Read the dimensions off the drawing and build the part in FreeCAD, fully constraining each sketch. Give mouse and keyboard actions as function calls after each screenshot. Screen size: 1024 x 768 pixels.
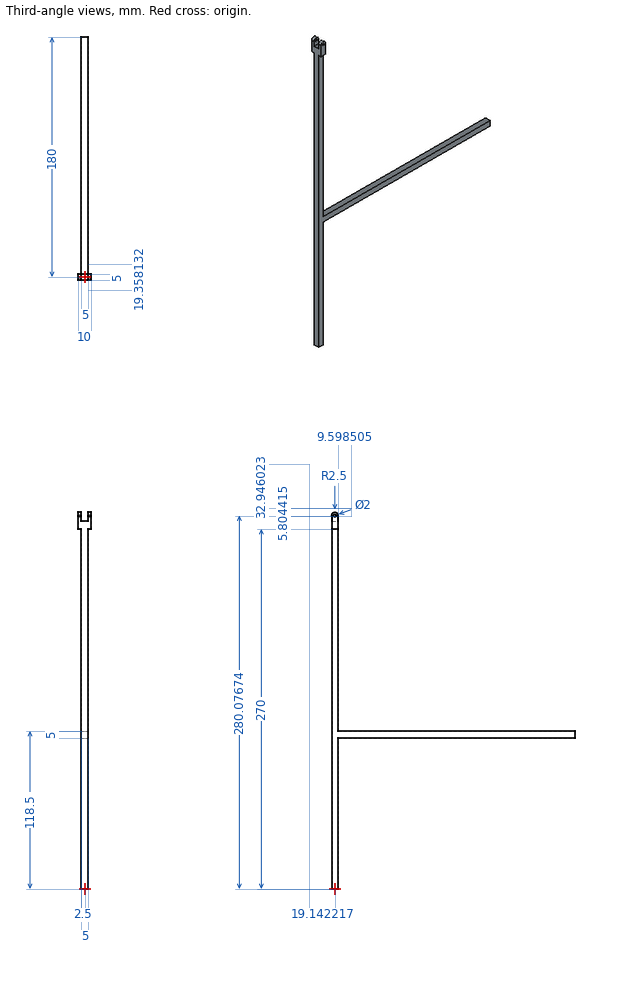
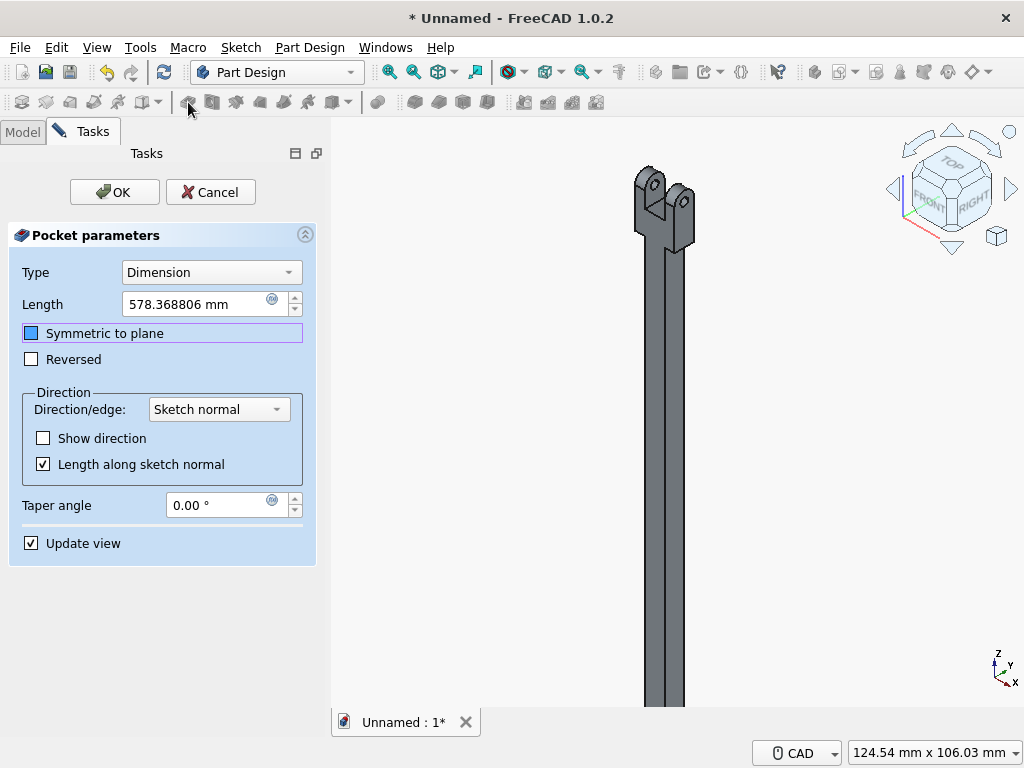
click(30, 333)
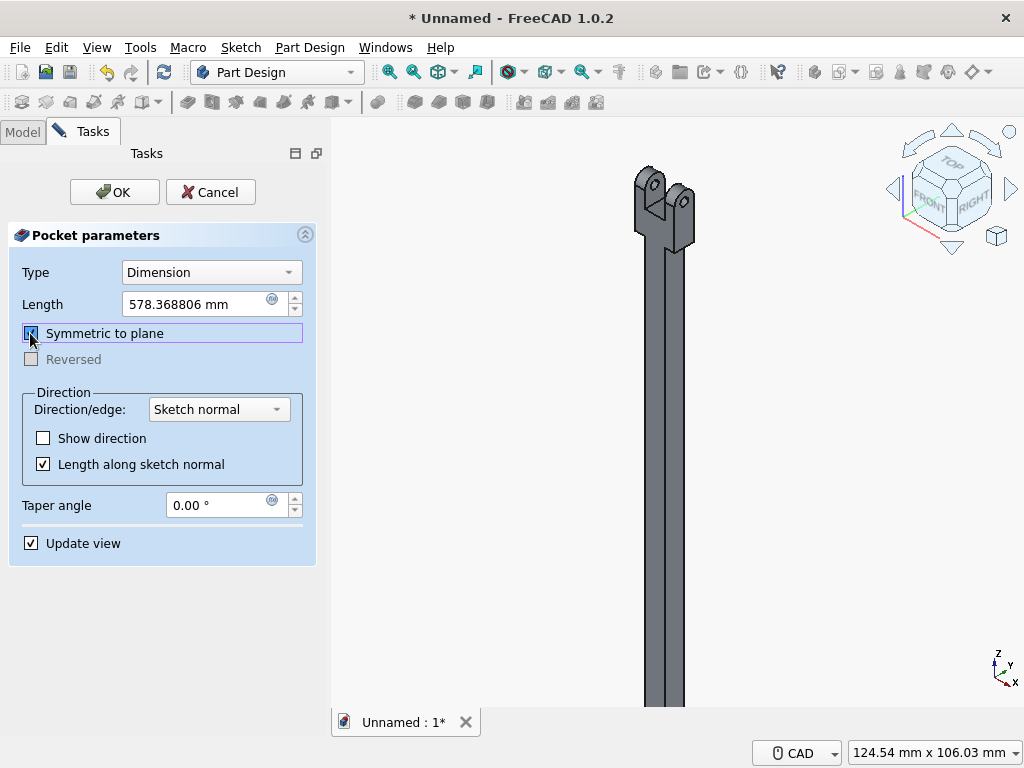
click(115, 192)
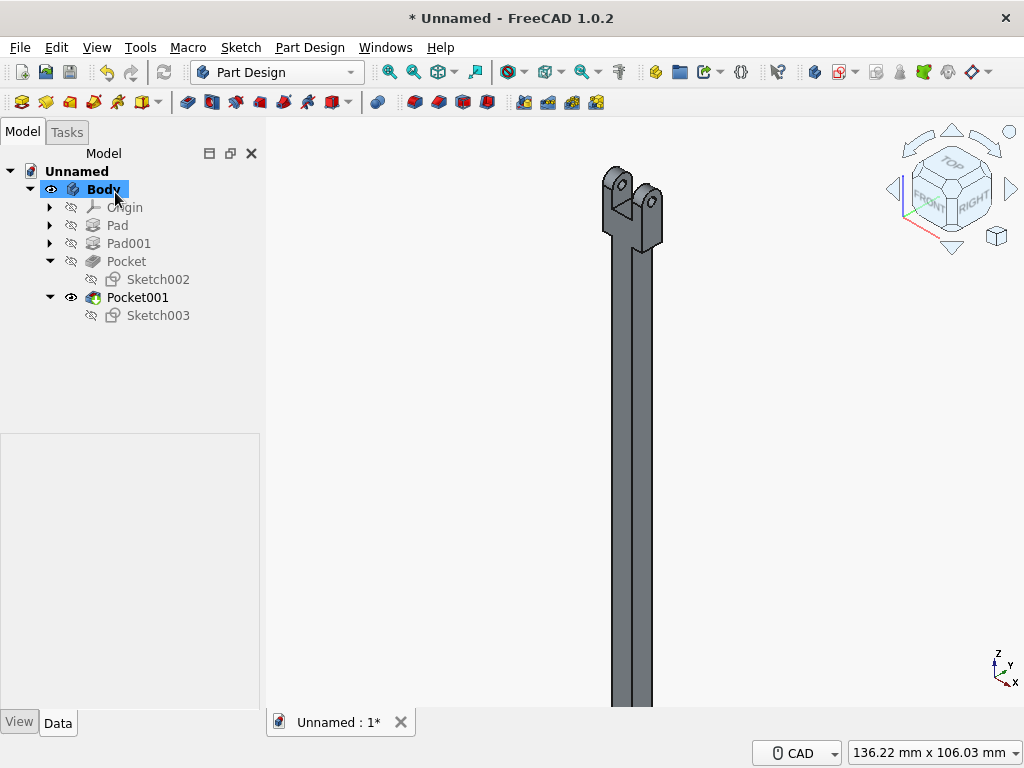
click(390, 72)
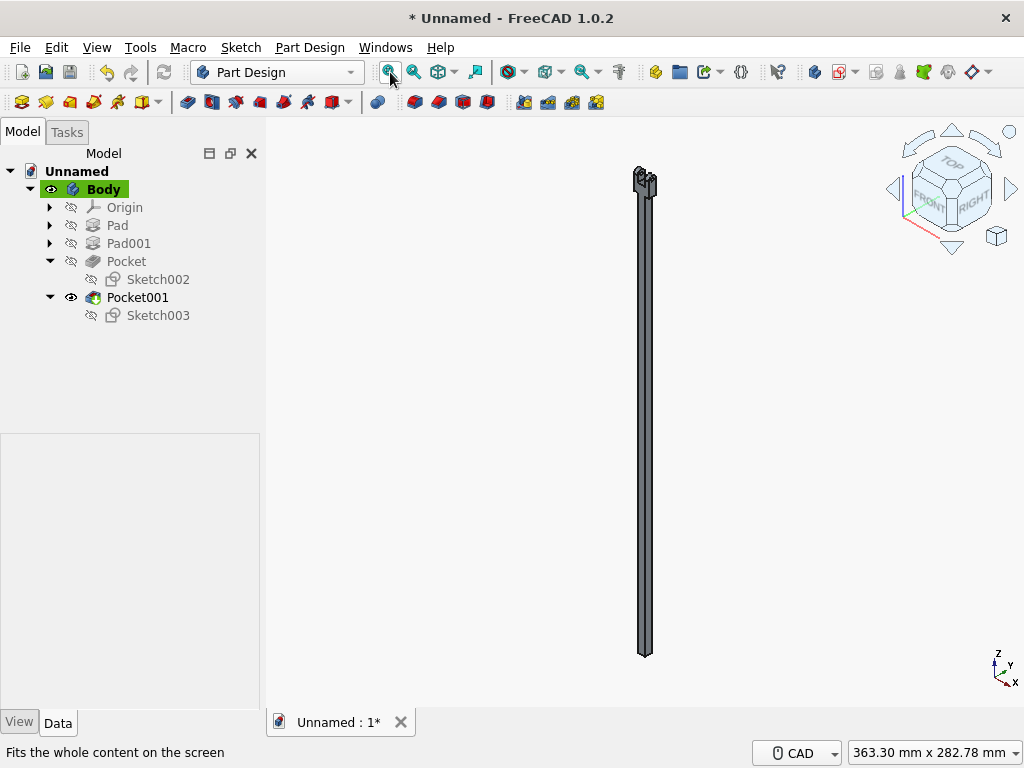
click(840, 72)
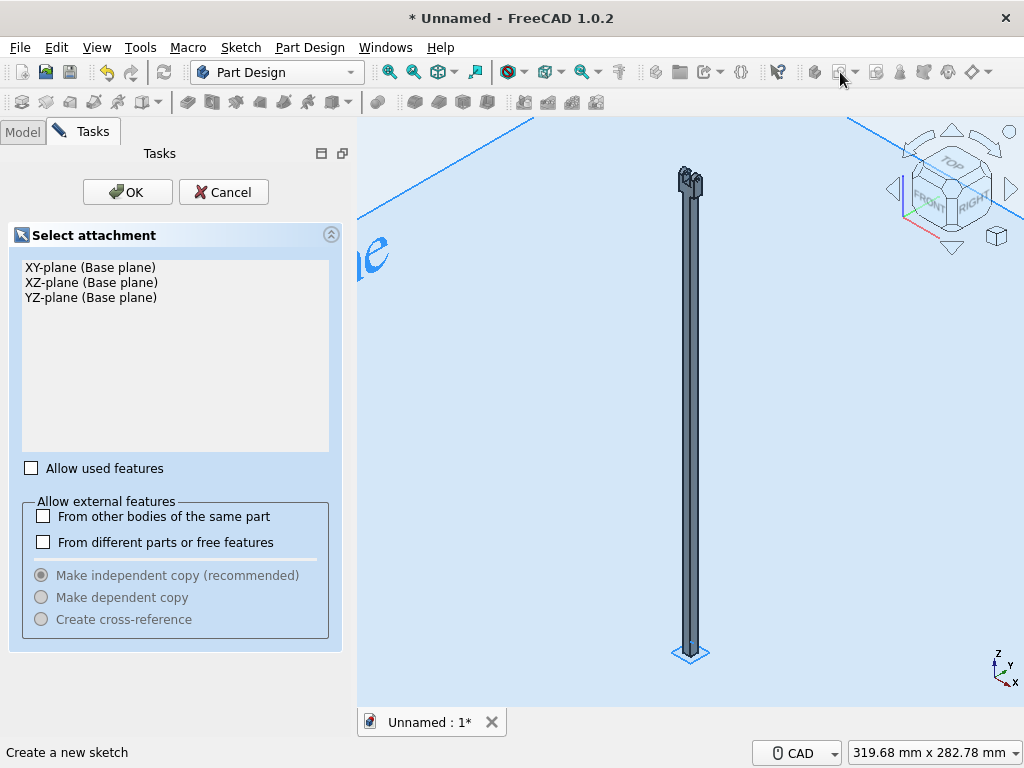
click(82, 282)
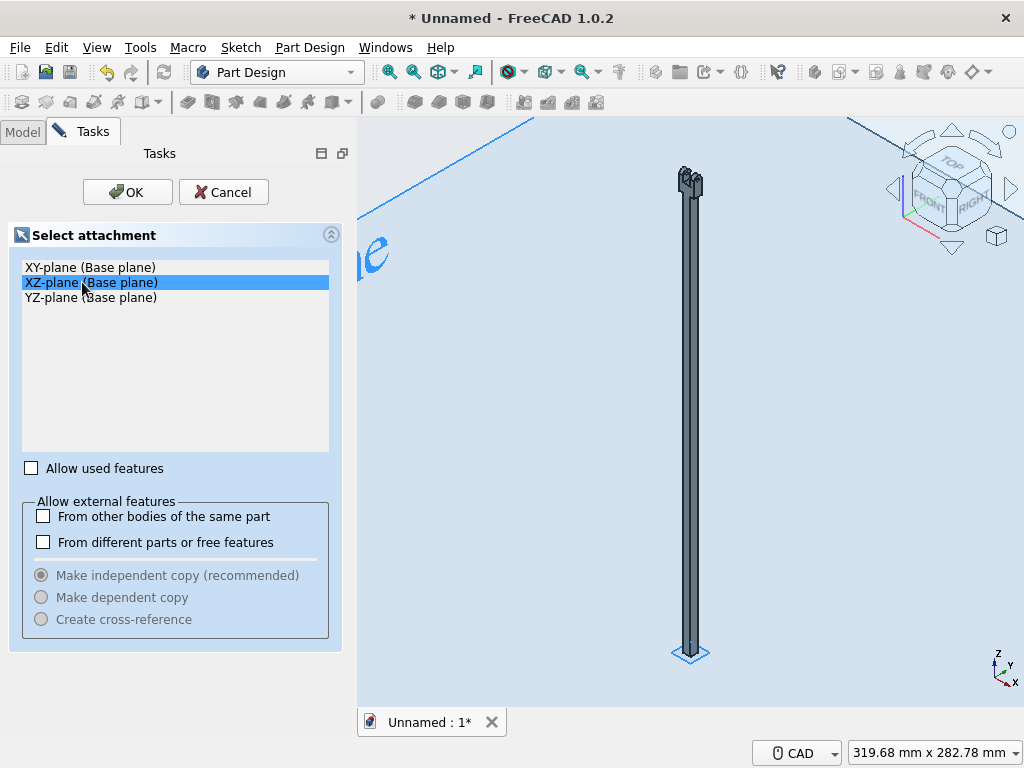
click(128, 192)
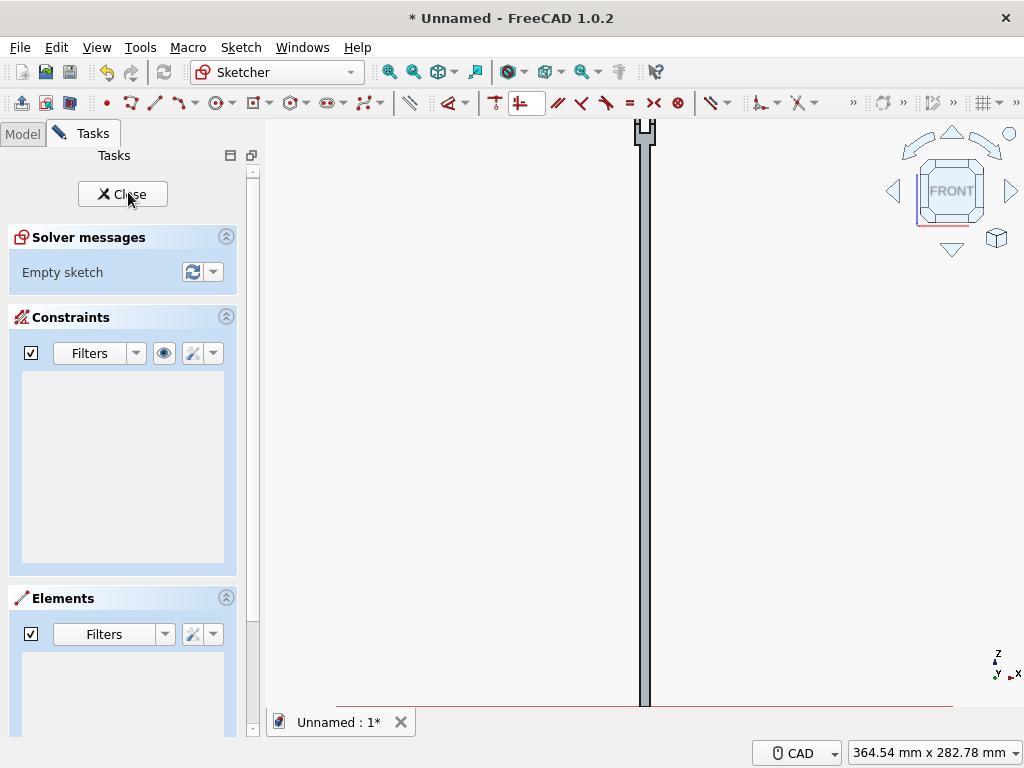
click(70, 104)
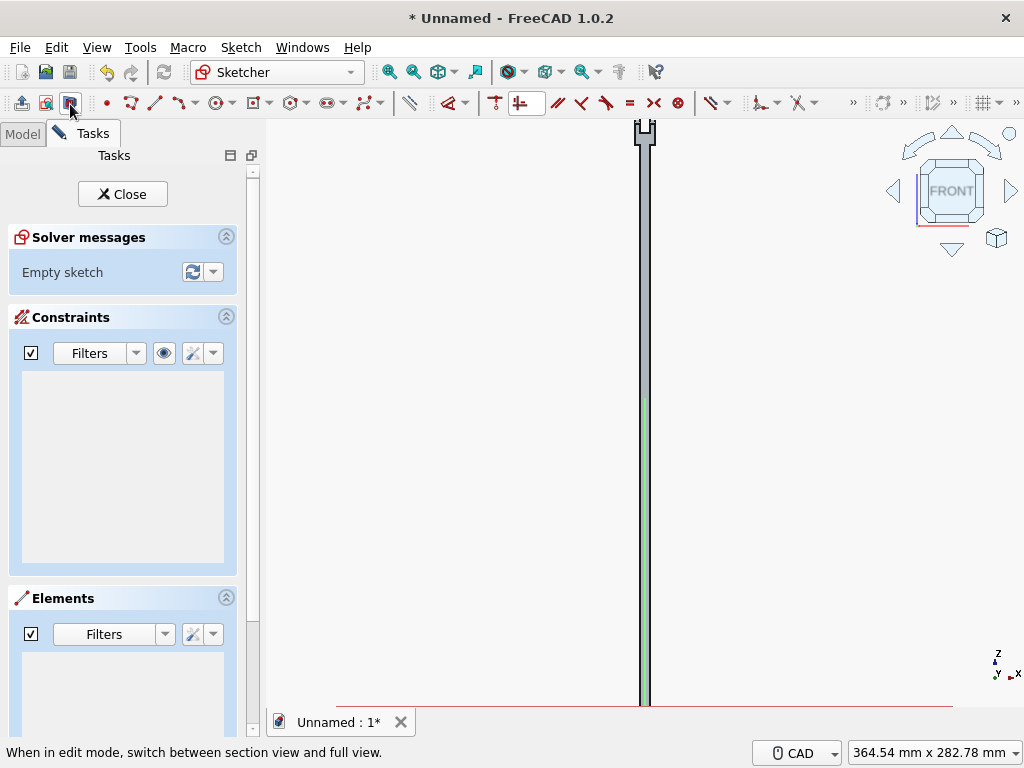
scroll(649, 468, up, 15)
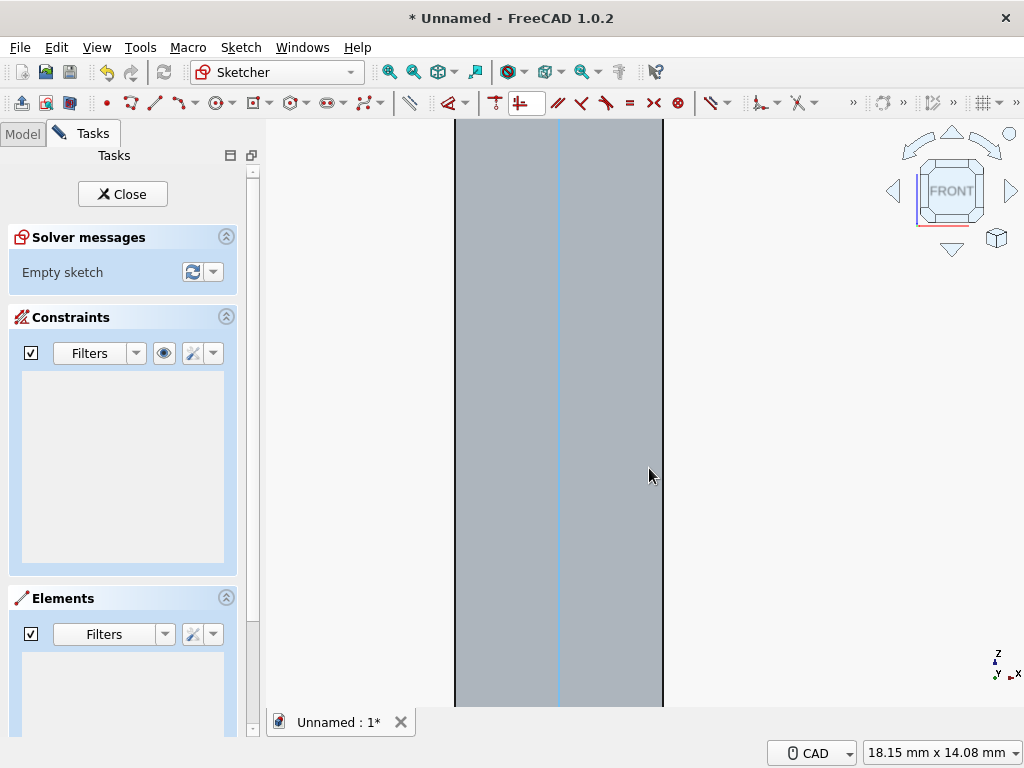
scroll(538, 401, up, 3)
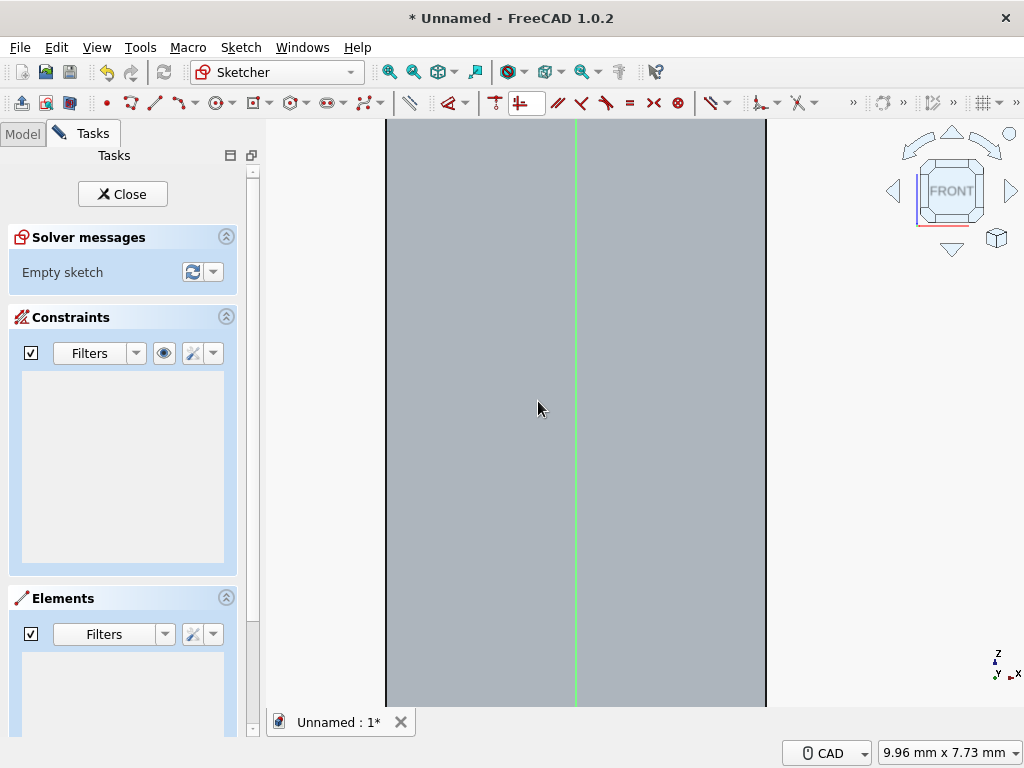
key(g)
key(r)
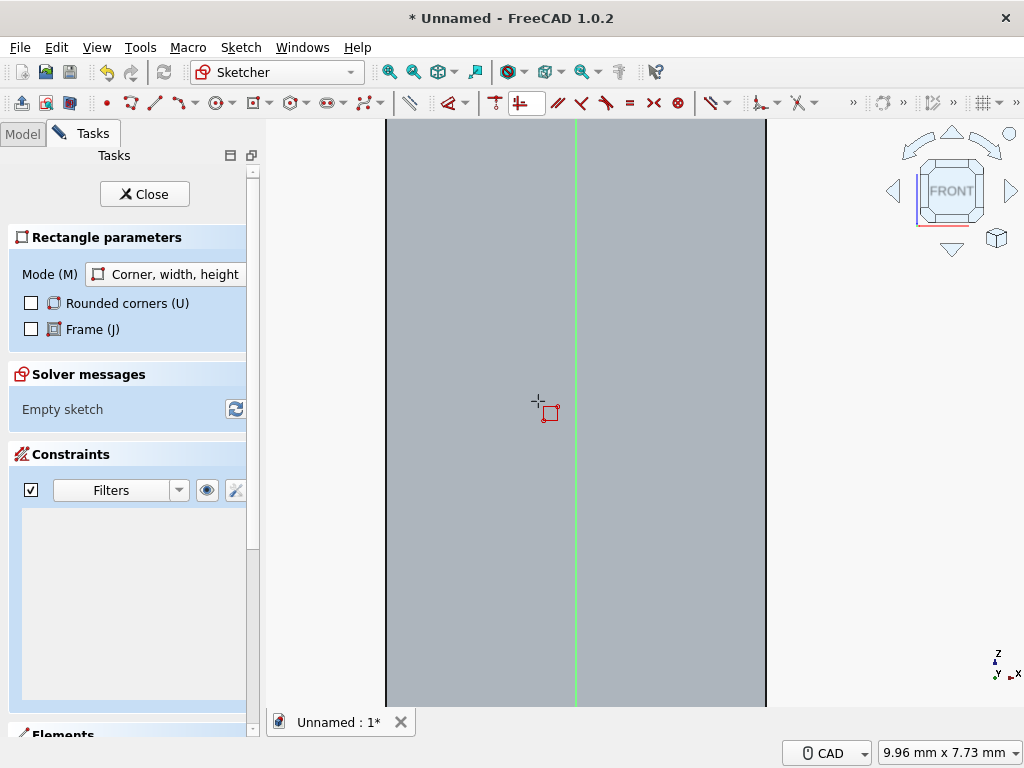
click(386, 223)
click(766, 603)
key(Escape)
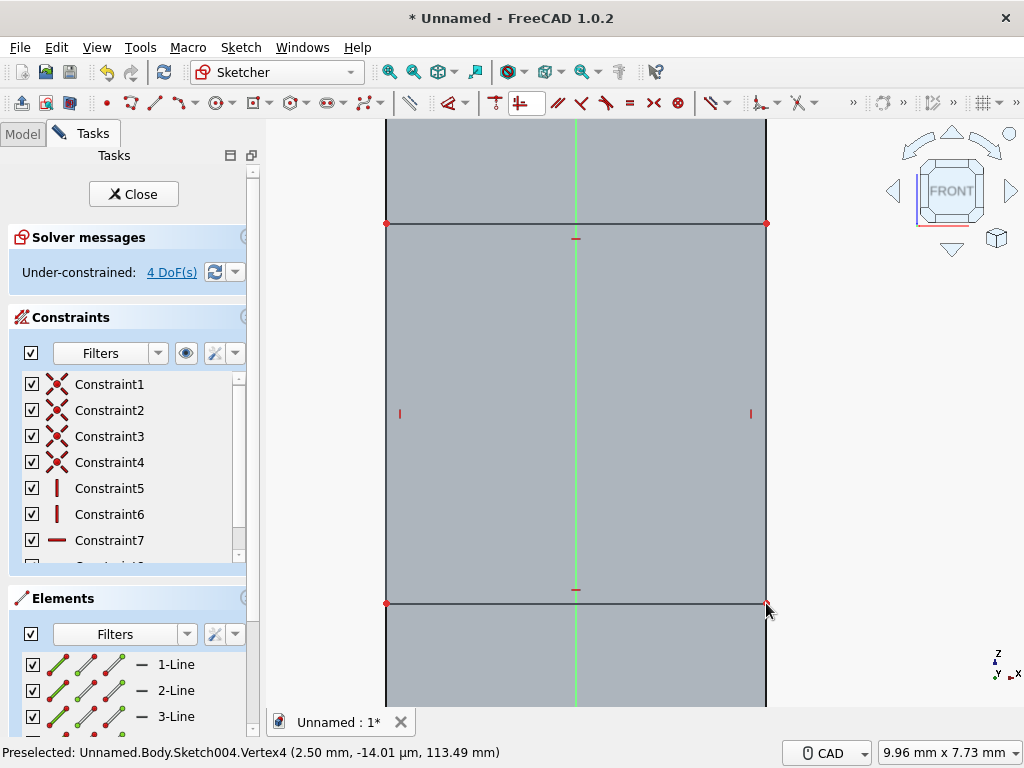
click(448, 104)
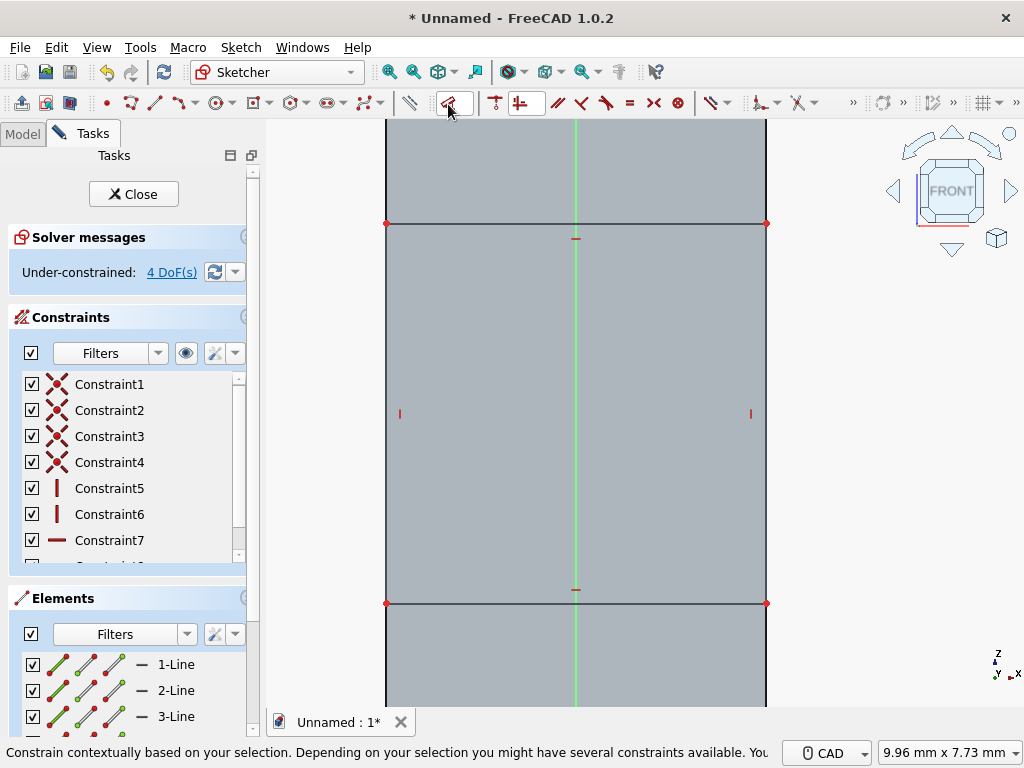
click(386, 338)
click(352, 414)